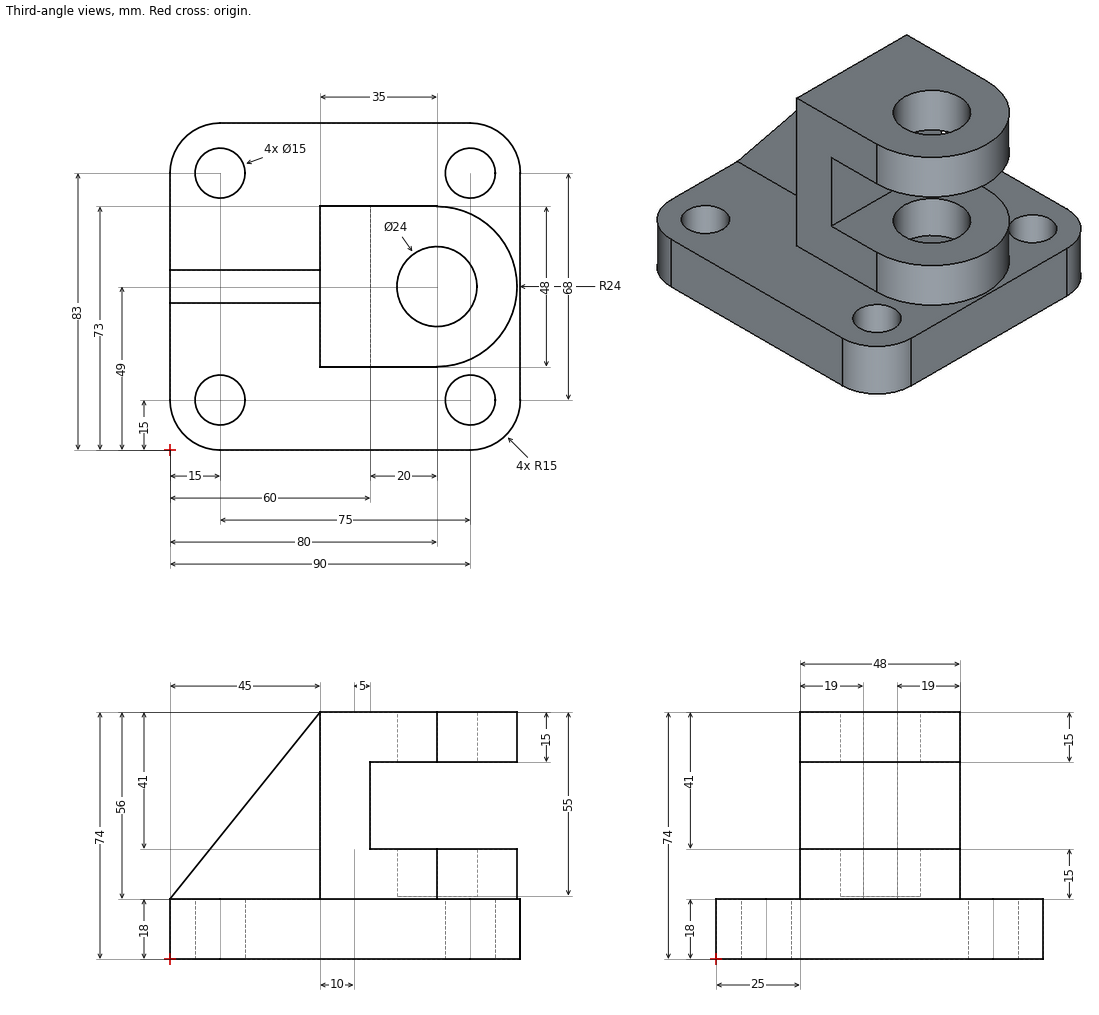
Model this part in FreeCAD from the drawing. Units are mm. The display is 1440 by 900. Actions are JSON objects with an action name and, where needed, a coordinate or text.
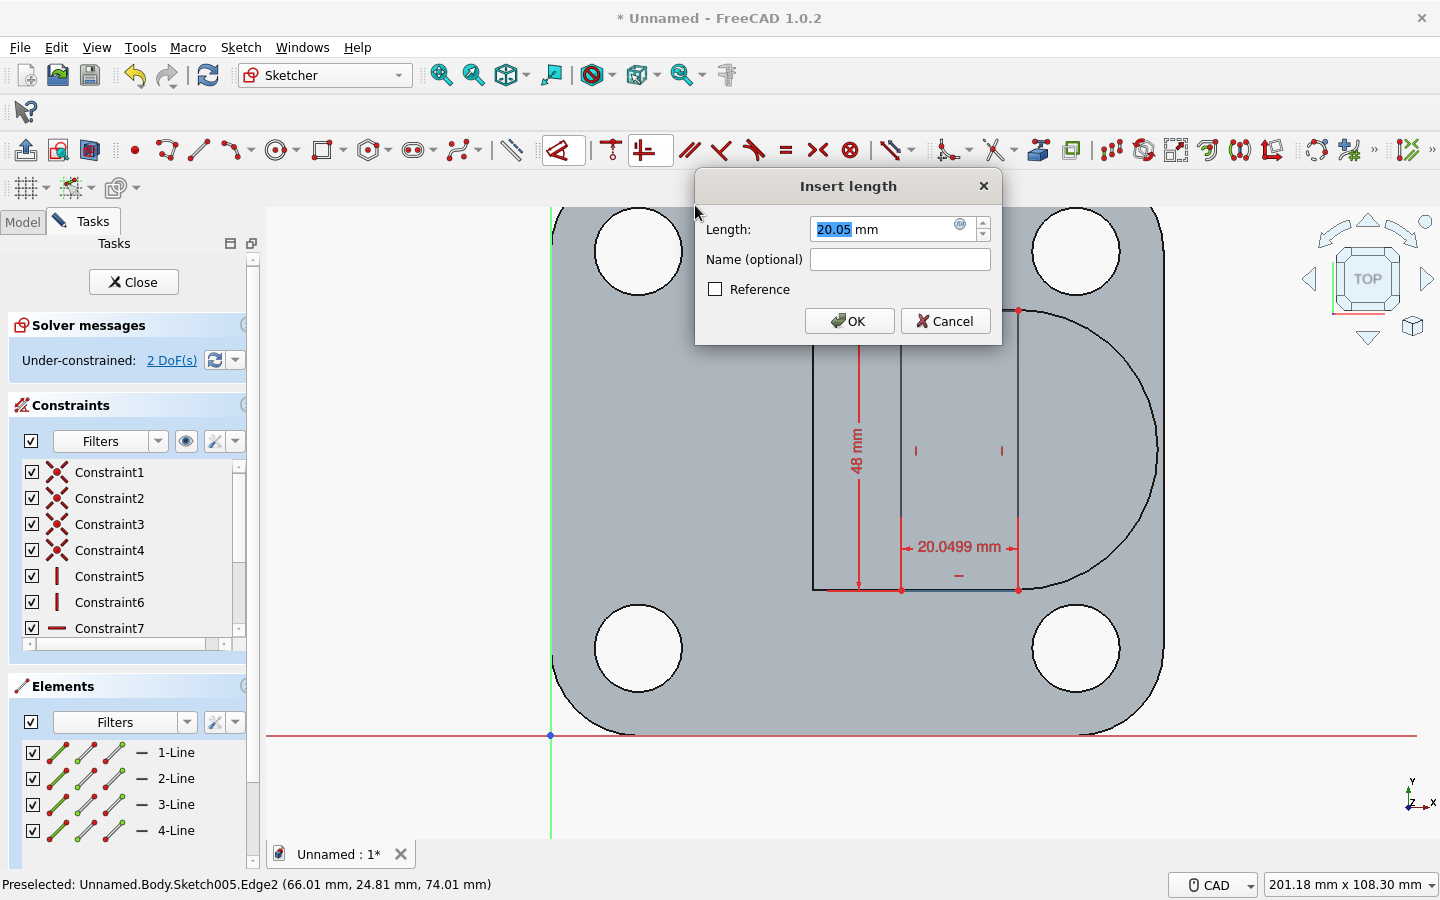
{"action": "type", "text": "20"}
{"action": "key", "text": "Return"}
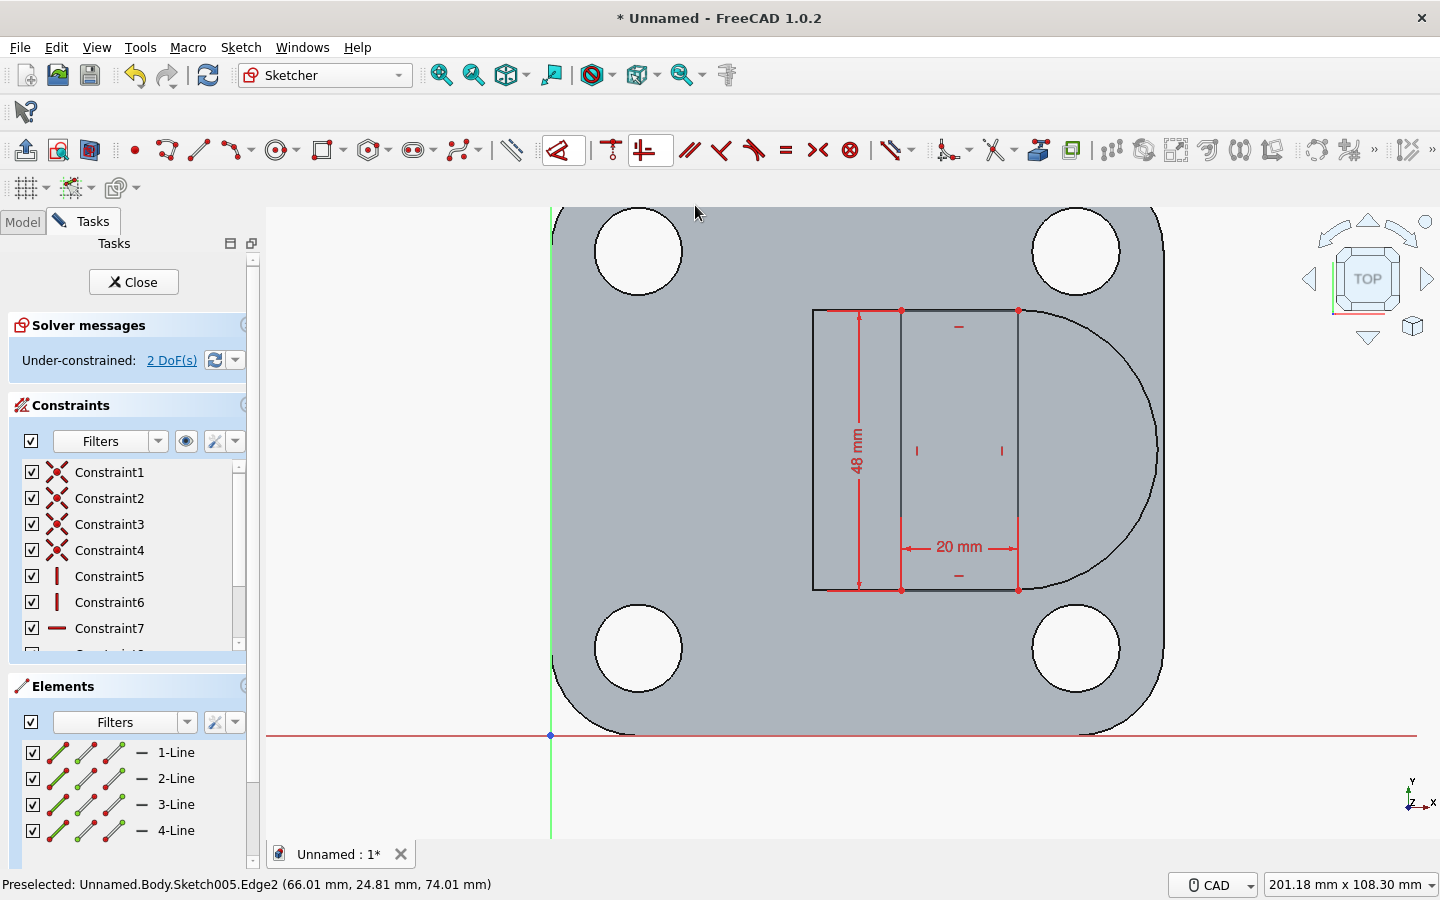
{"action": "left_click", "coordinate": [901, 311]}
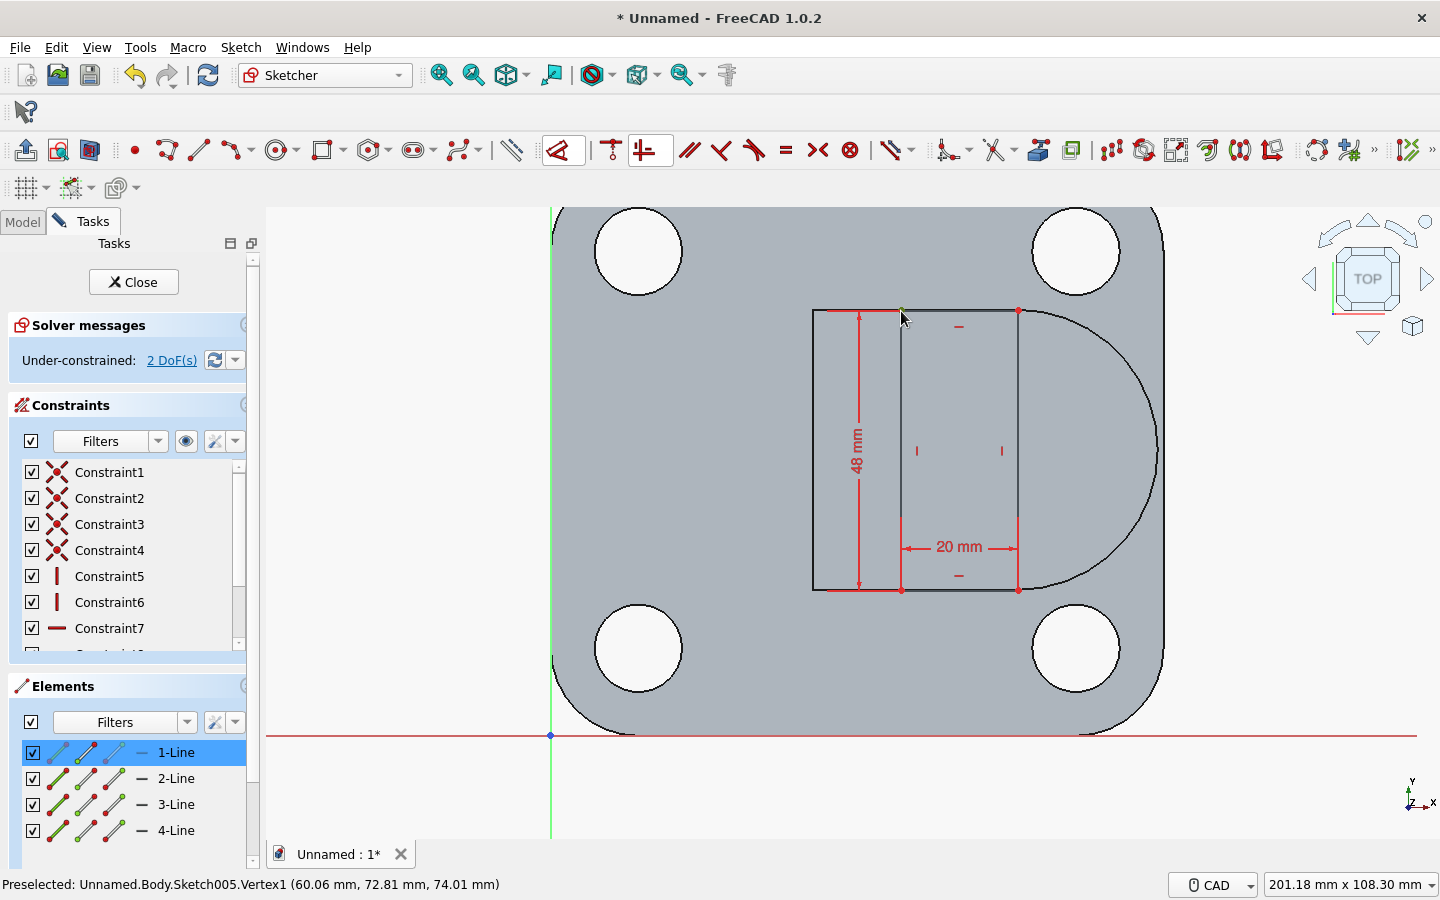
{"action": "left_click", "coordinate": [580, 150]}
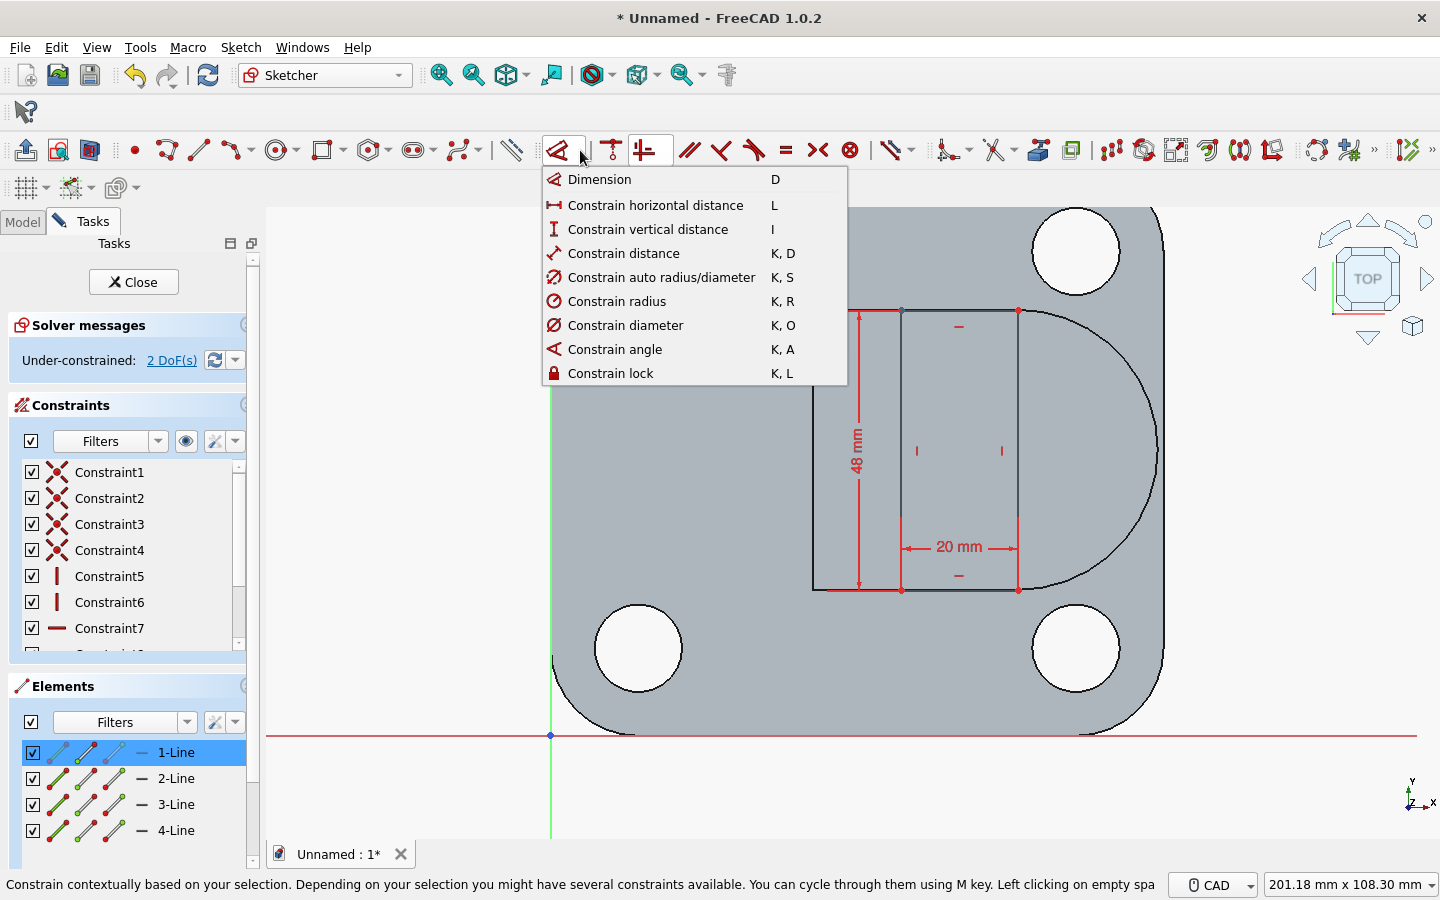
{"action": "left_click", "coordinate": [695, 205]}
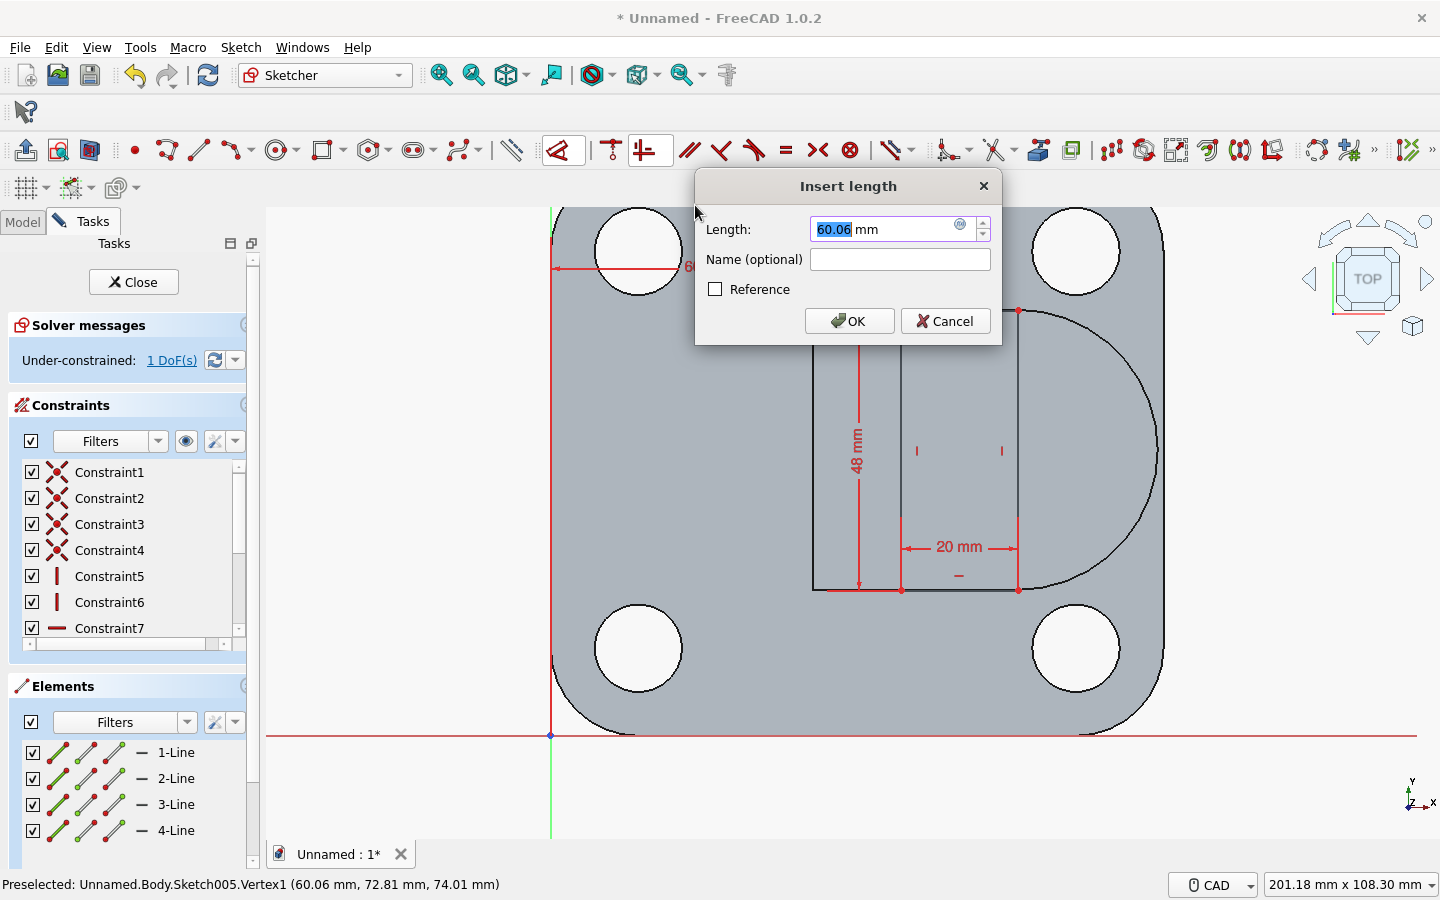
{"action": "type", "text": "60"}
{"action": "key", "text": "Return"}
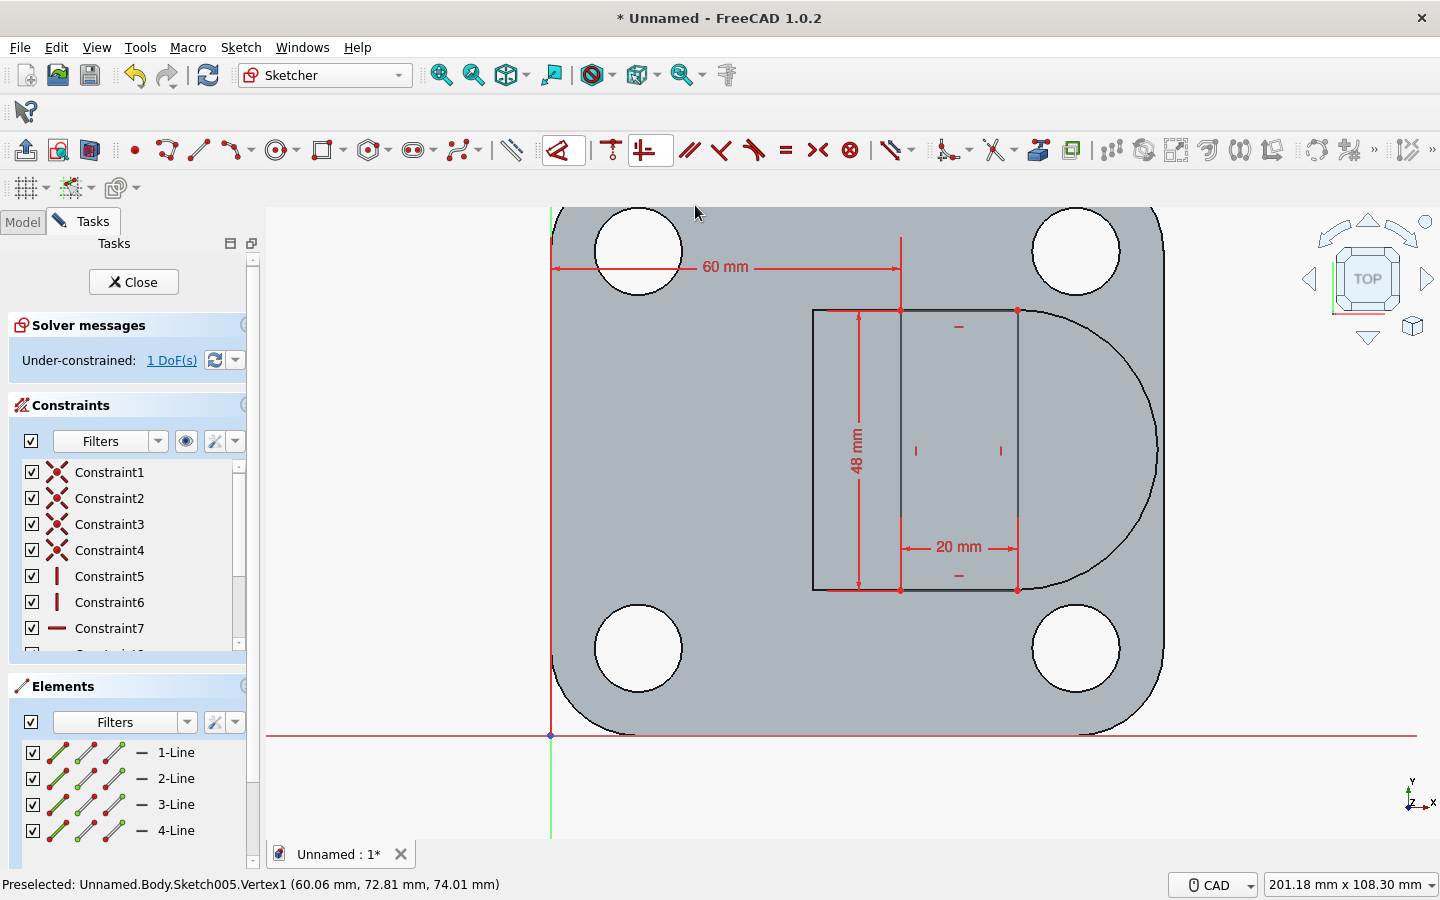
{"action": "left_click", "coordinate": [901, 311]}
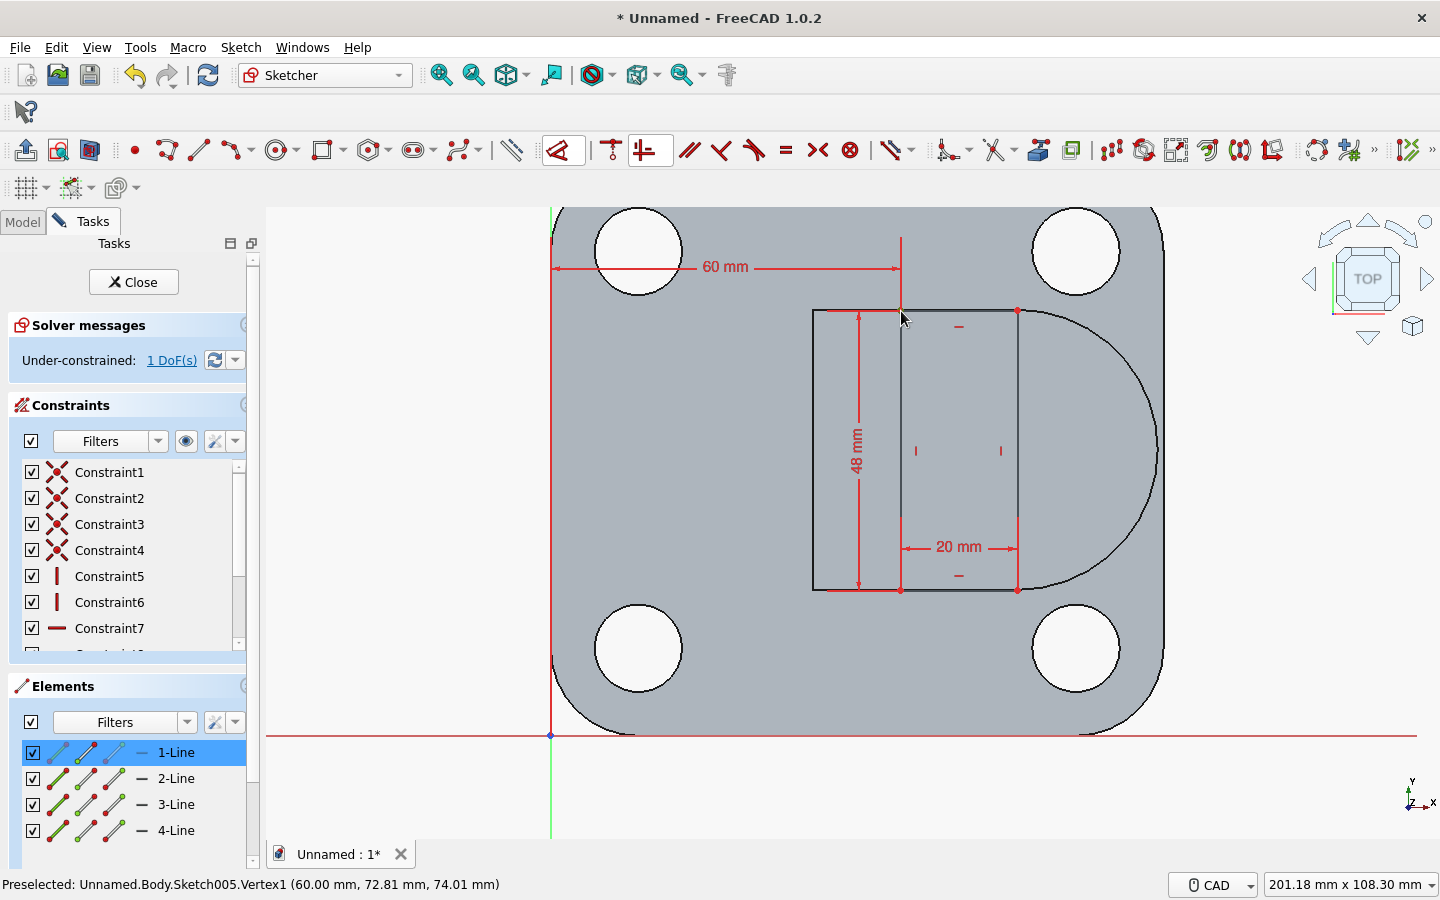
{"action": "key", "text": "i"}